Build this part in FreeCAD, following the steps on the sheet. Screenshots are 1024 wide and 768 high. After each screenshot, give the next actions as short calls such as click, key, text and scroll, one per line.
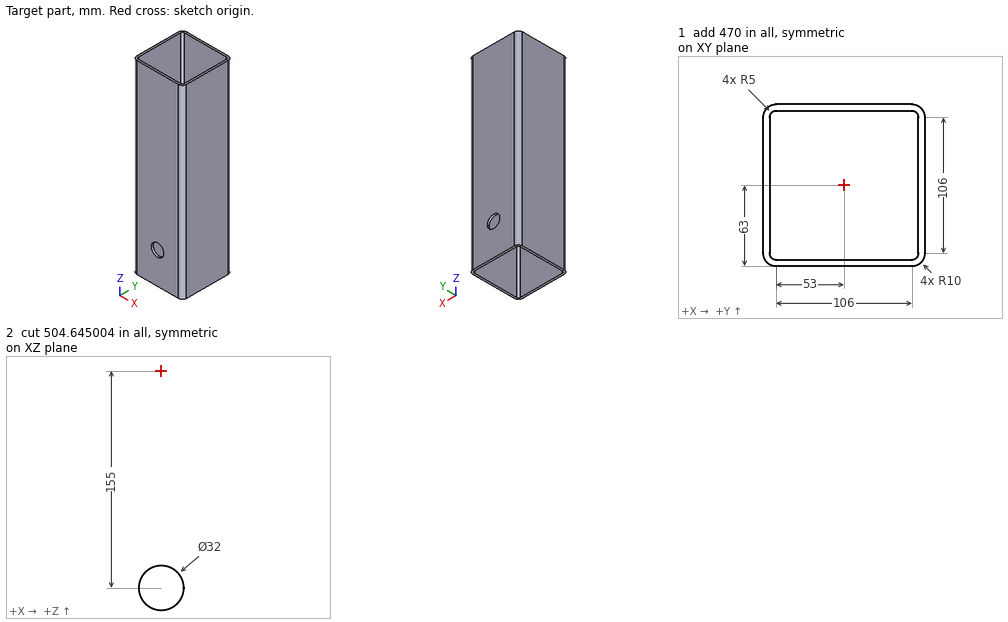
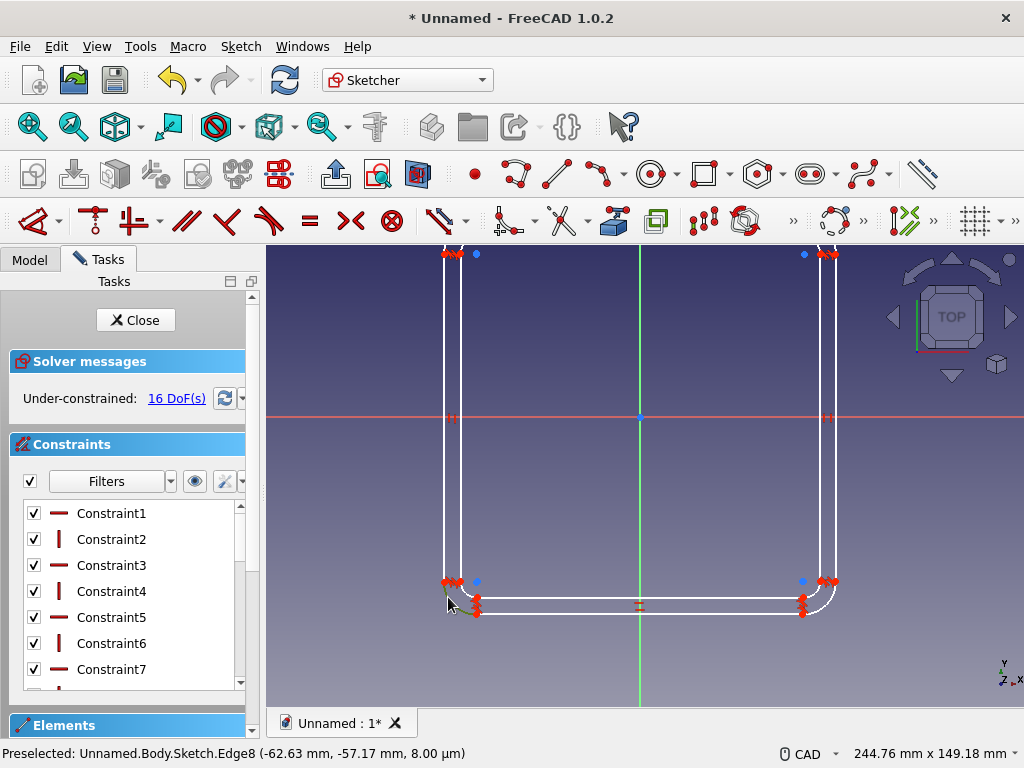
click(466, 593)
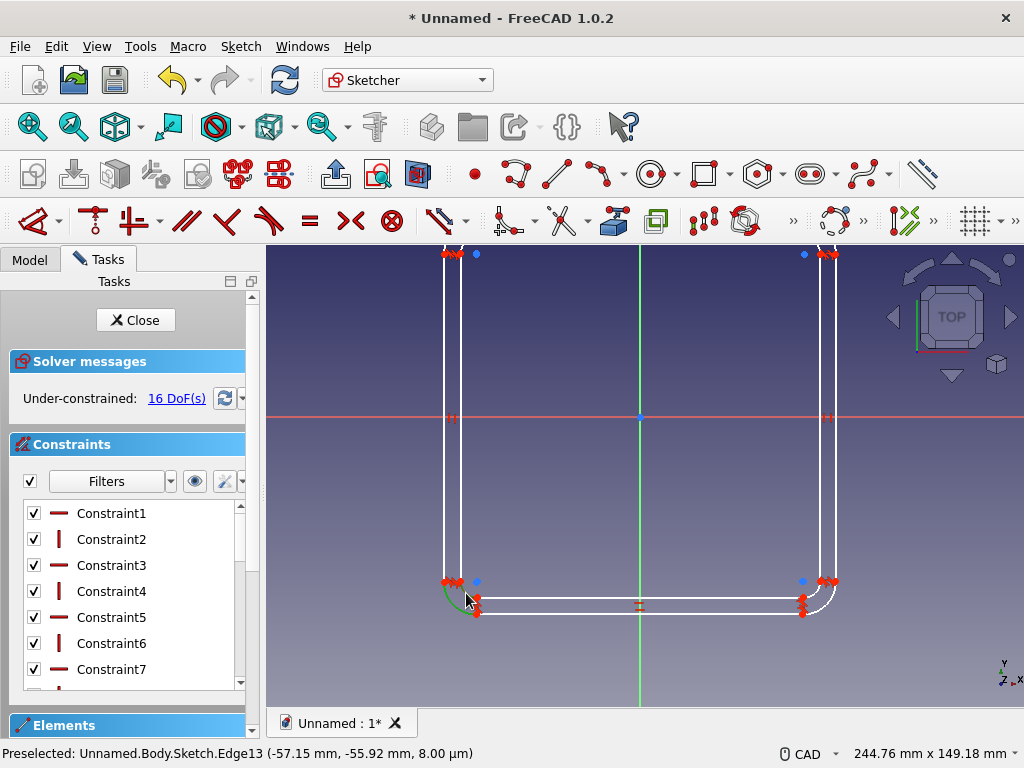
key(c)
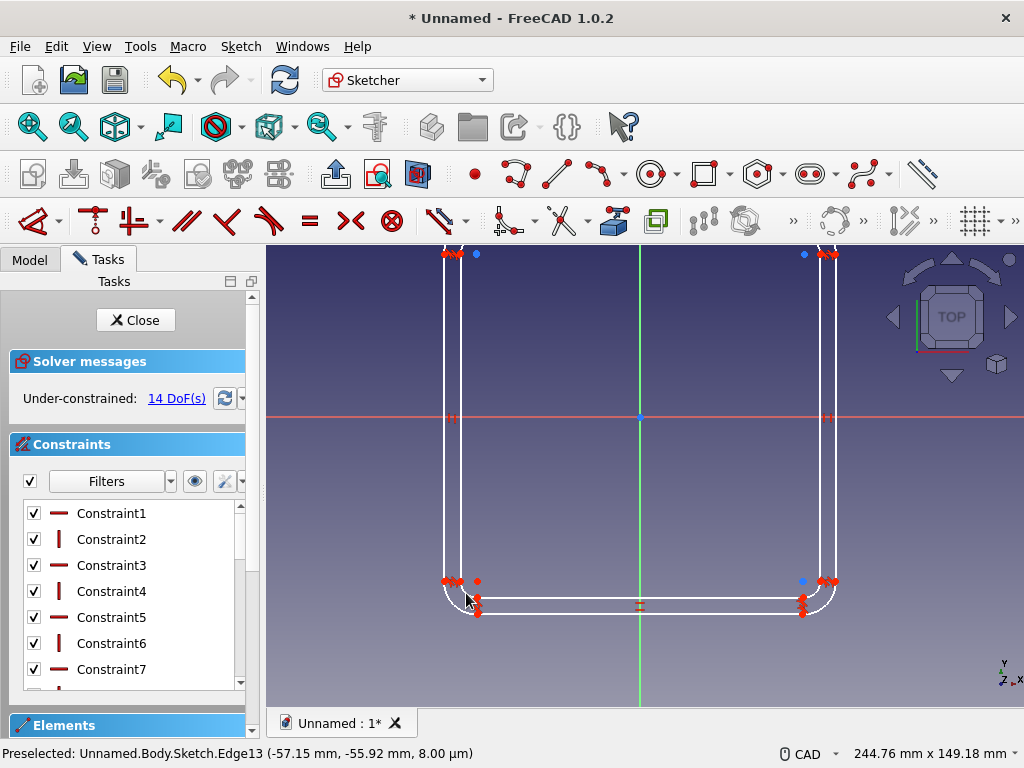
scroll(447, 596, down, 2)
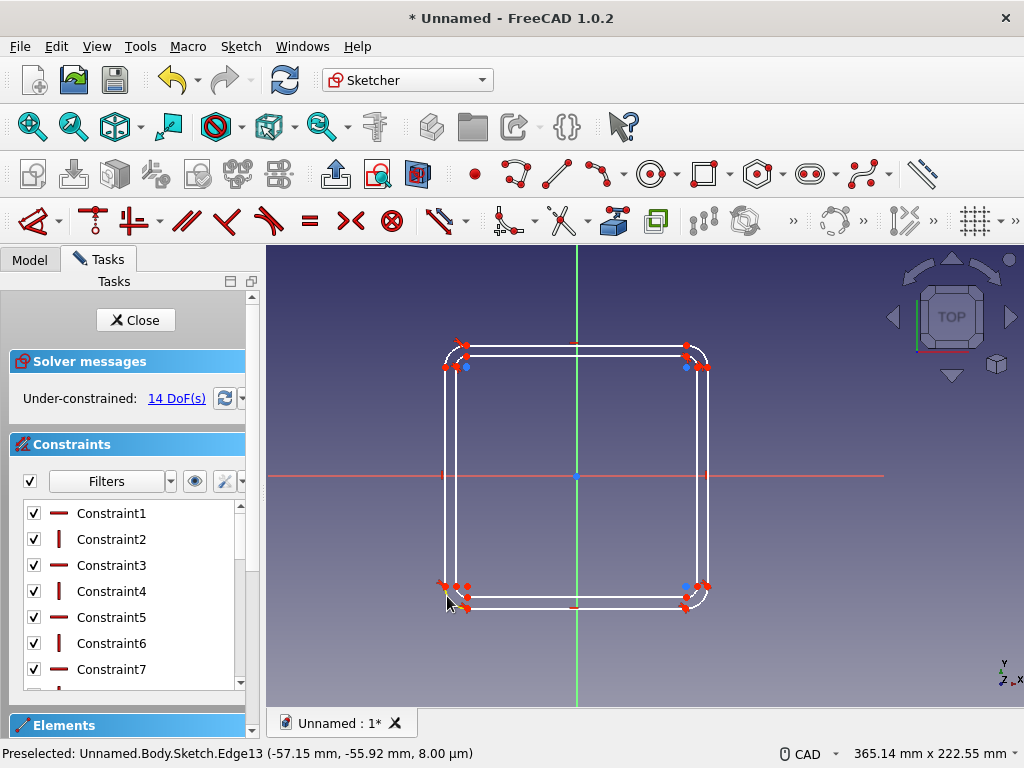
scroll(457, 348, up, 2)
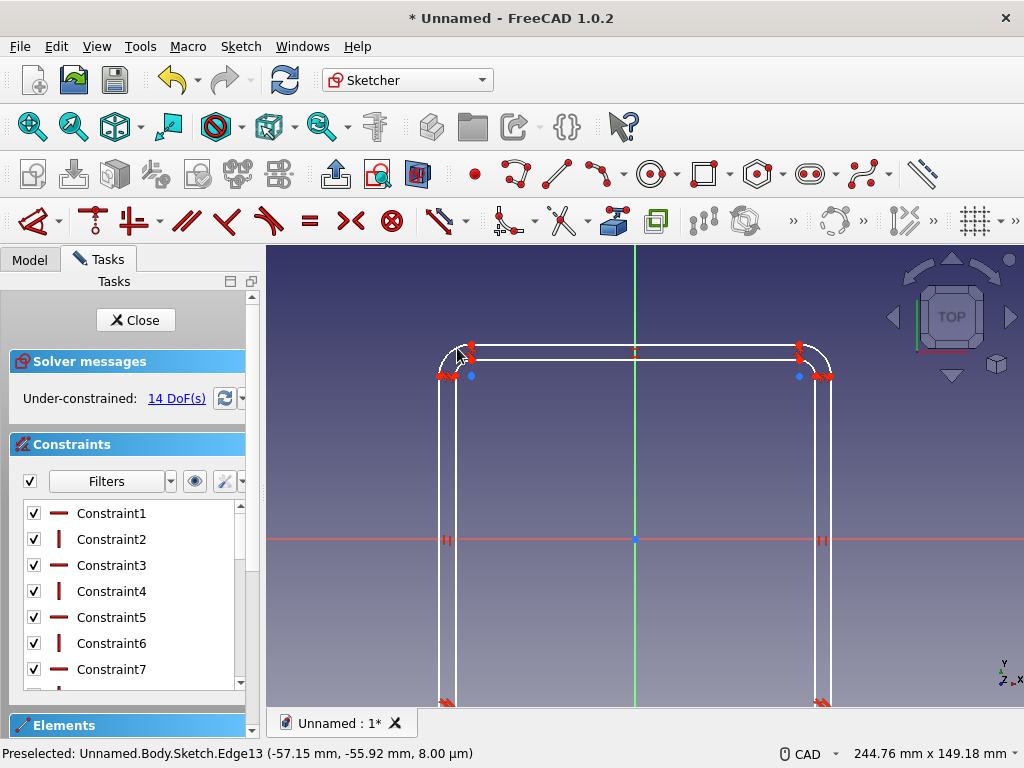
click(457, 348)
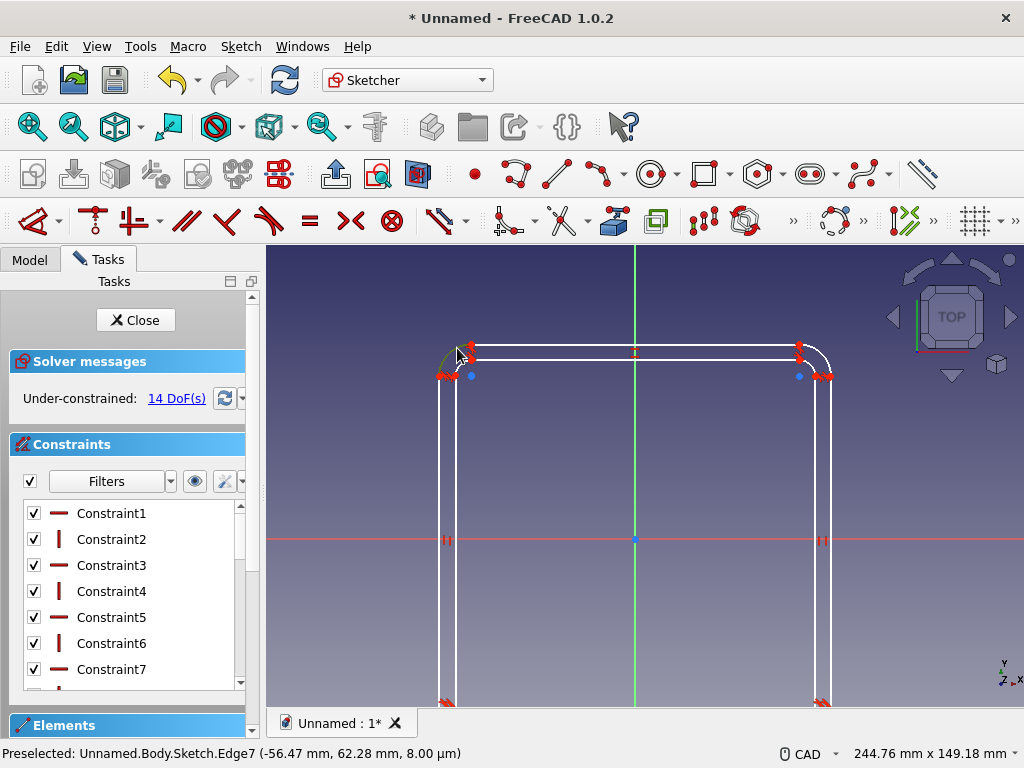
click(460, 365)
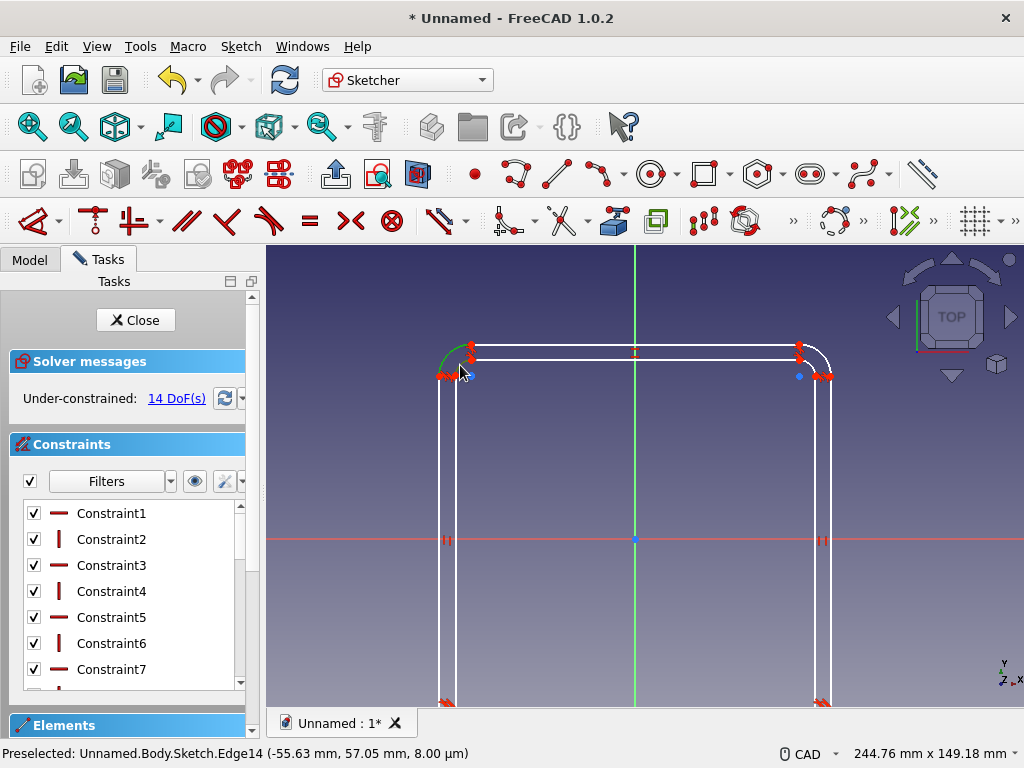
click(93, 222)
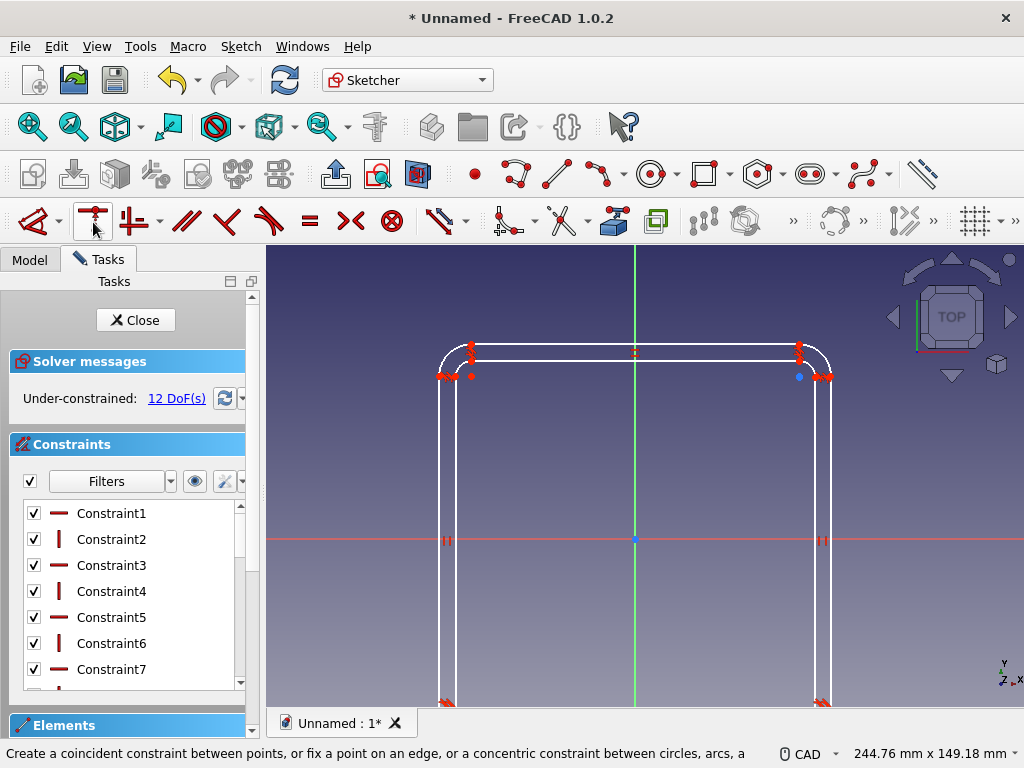
click(827, 362)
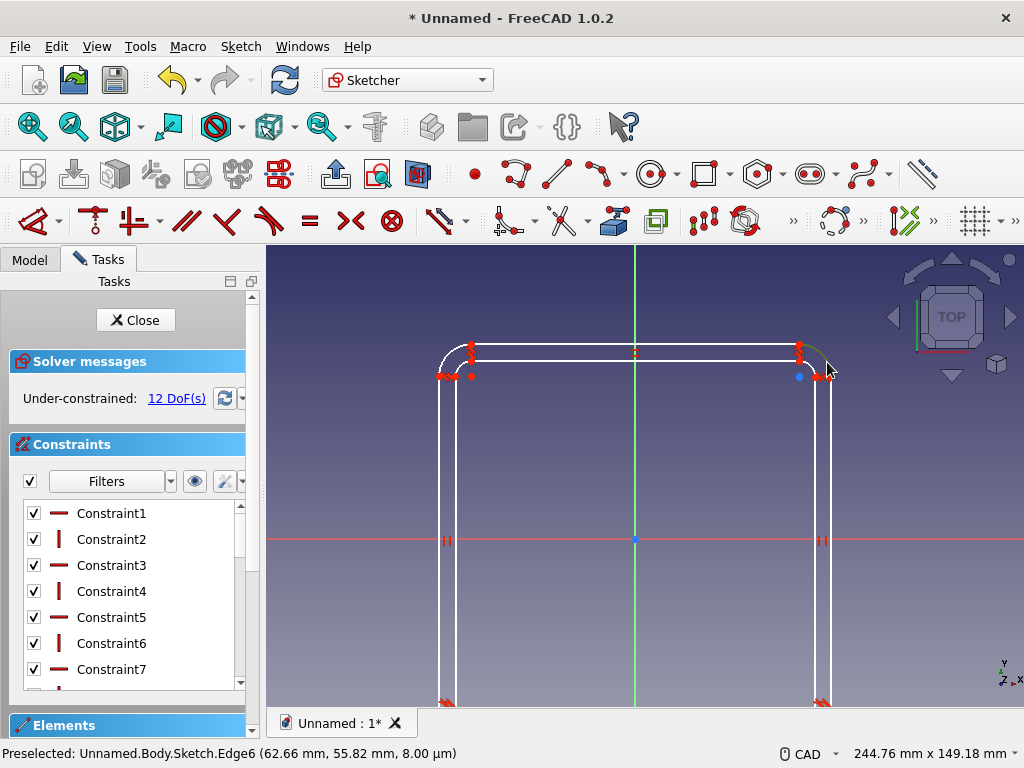
click(811, 366)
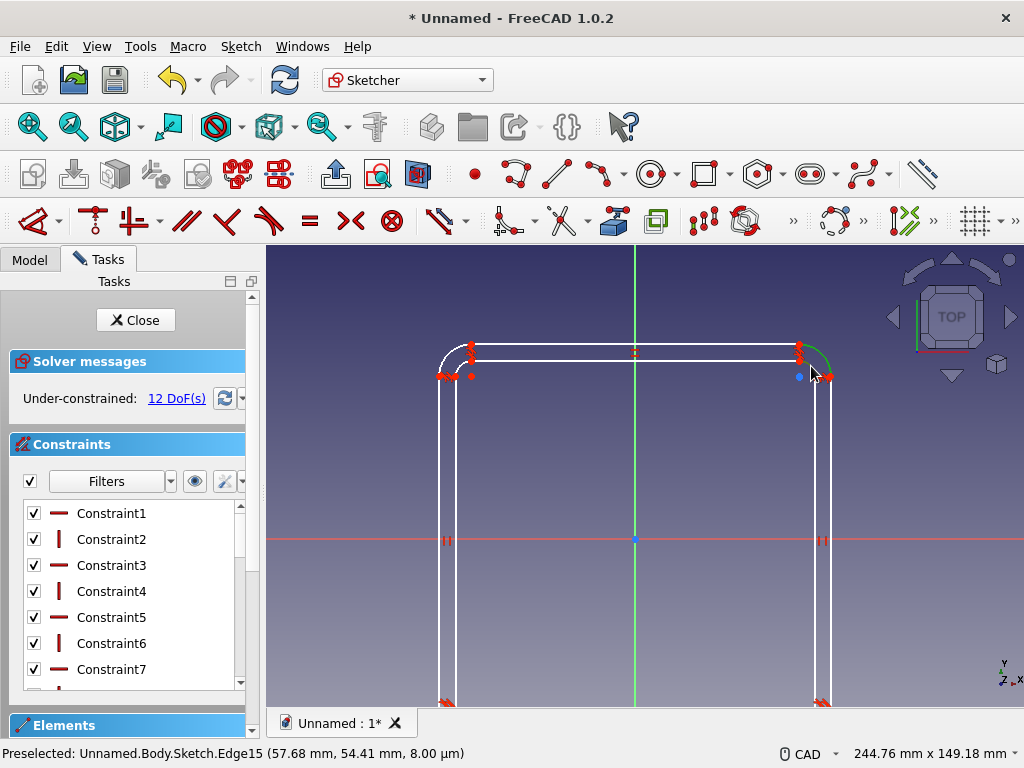
key(c)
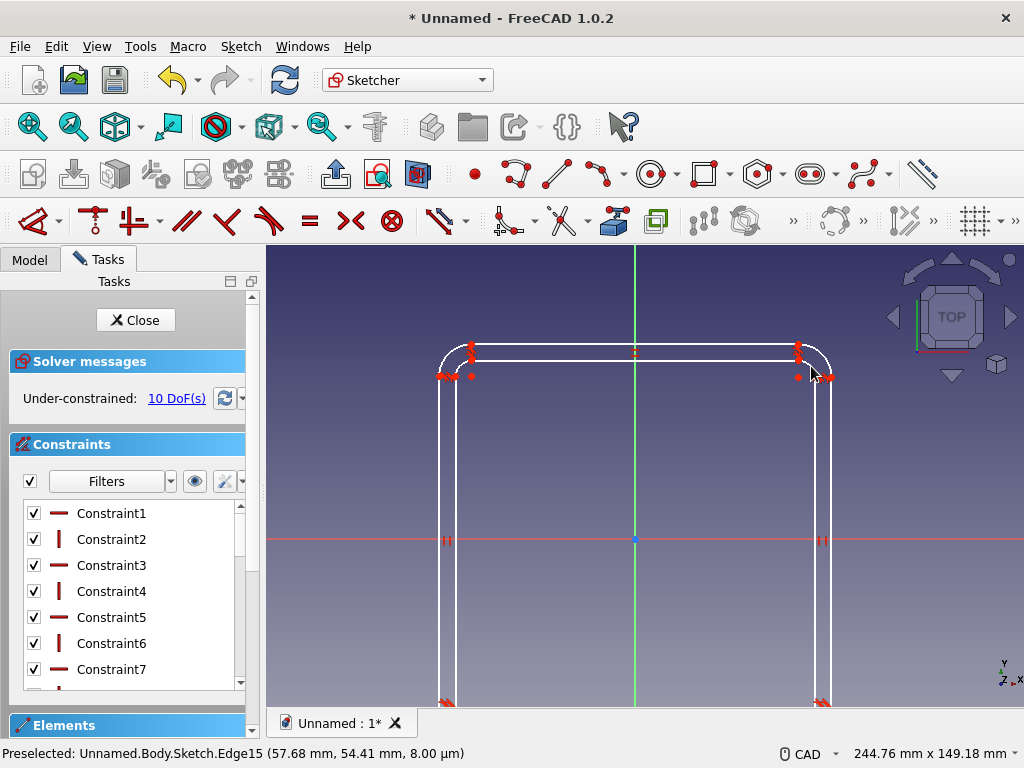
scroll(457, 347, down, 2)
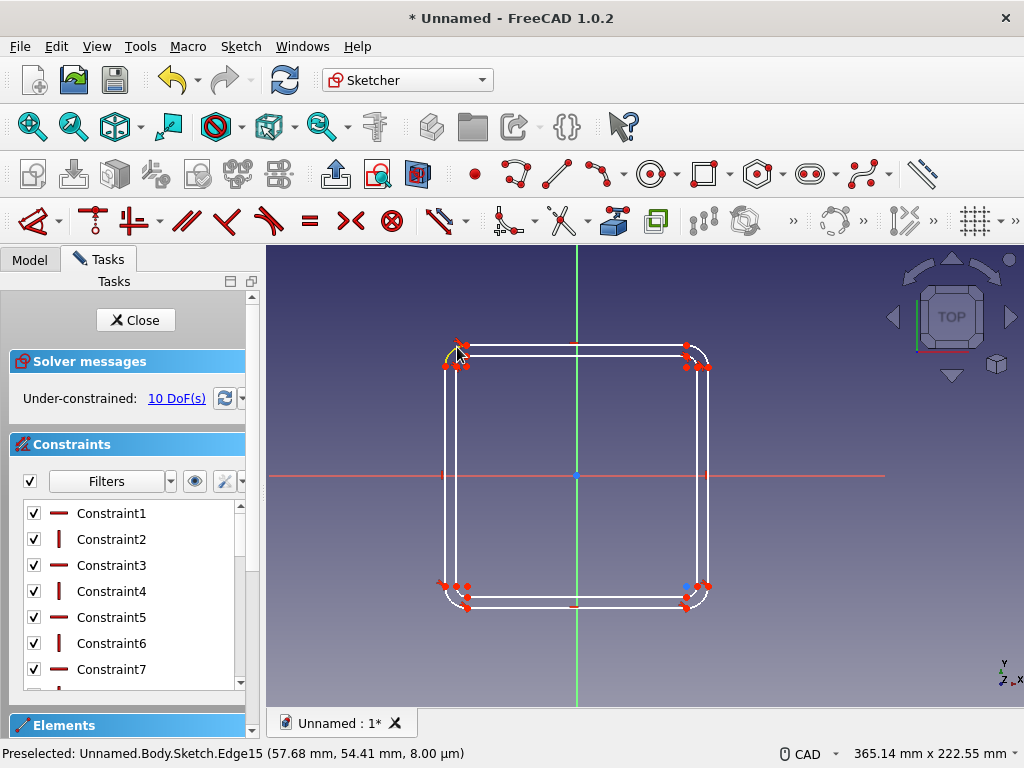
scroll(696, 606, up, 2)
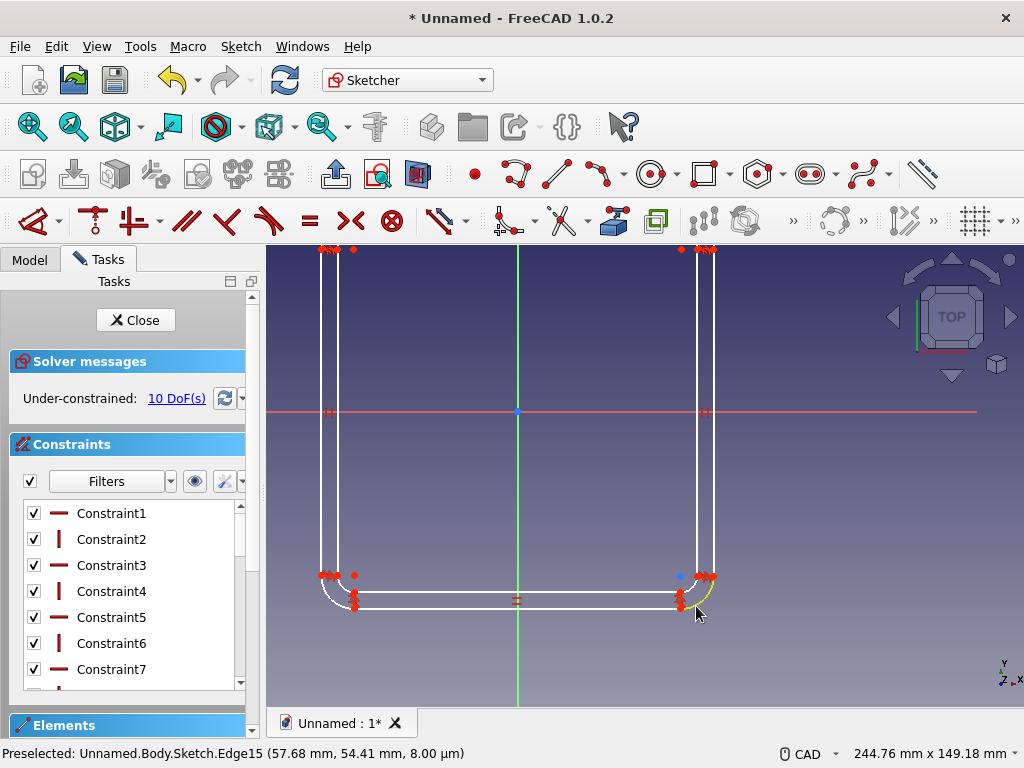
click(696, 605)